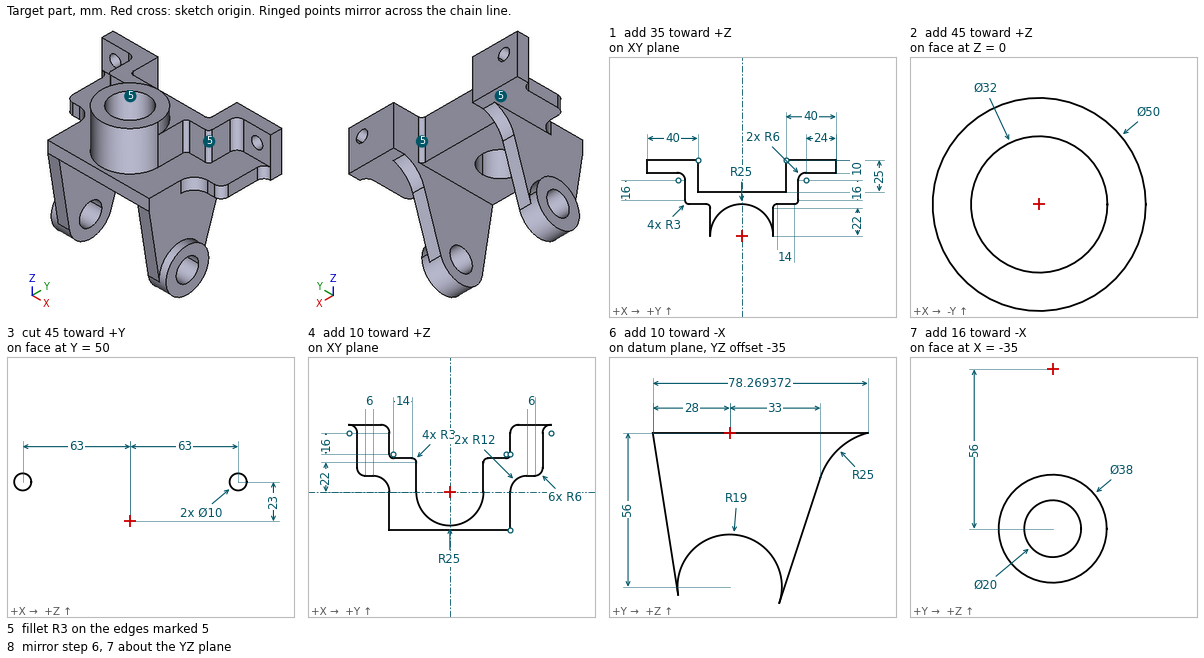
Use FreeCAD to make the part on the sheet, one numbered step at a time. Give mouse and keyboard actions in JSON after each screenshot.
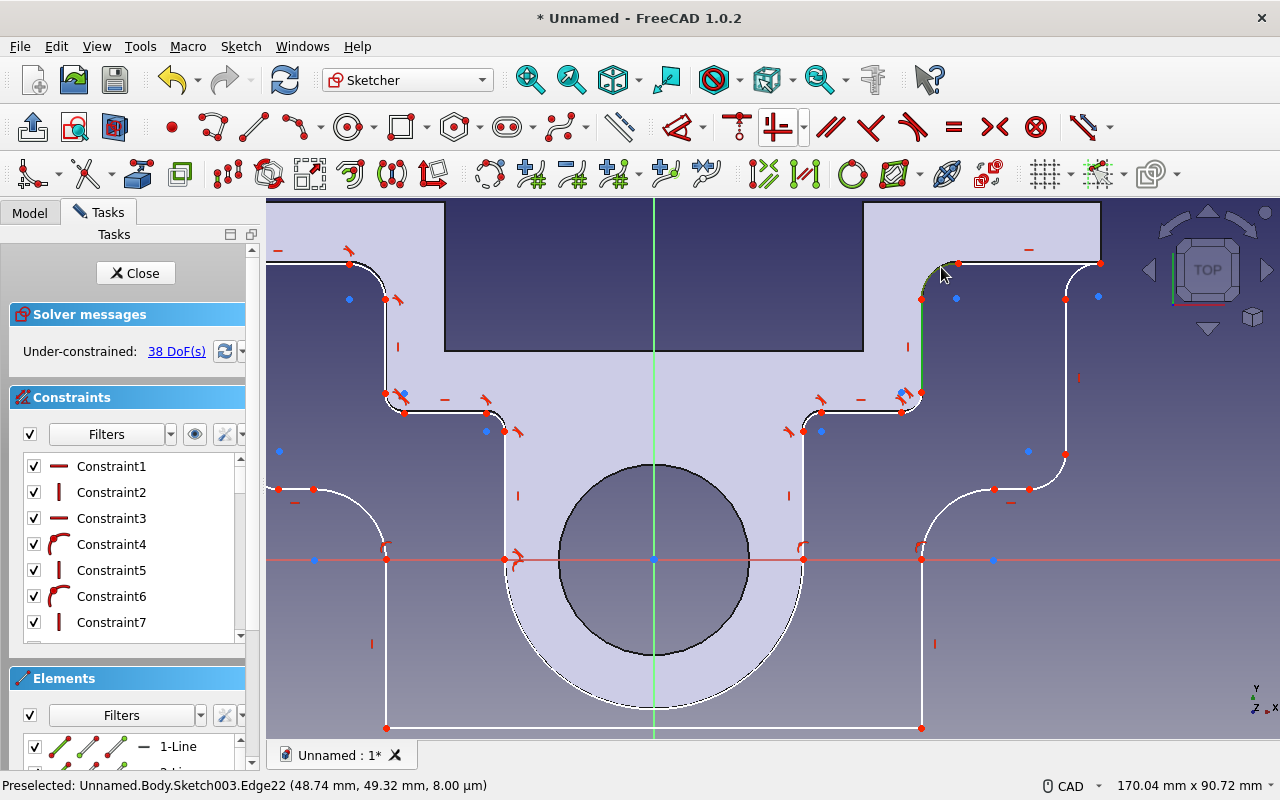
{"action": "left_click", "coordinate": [913, 128]}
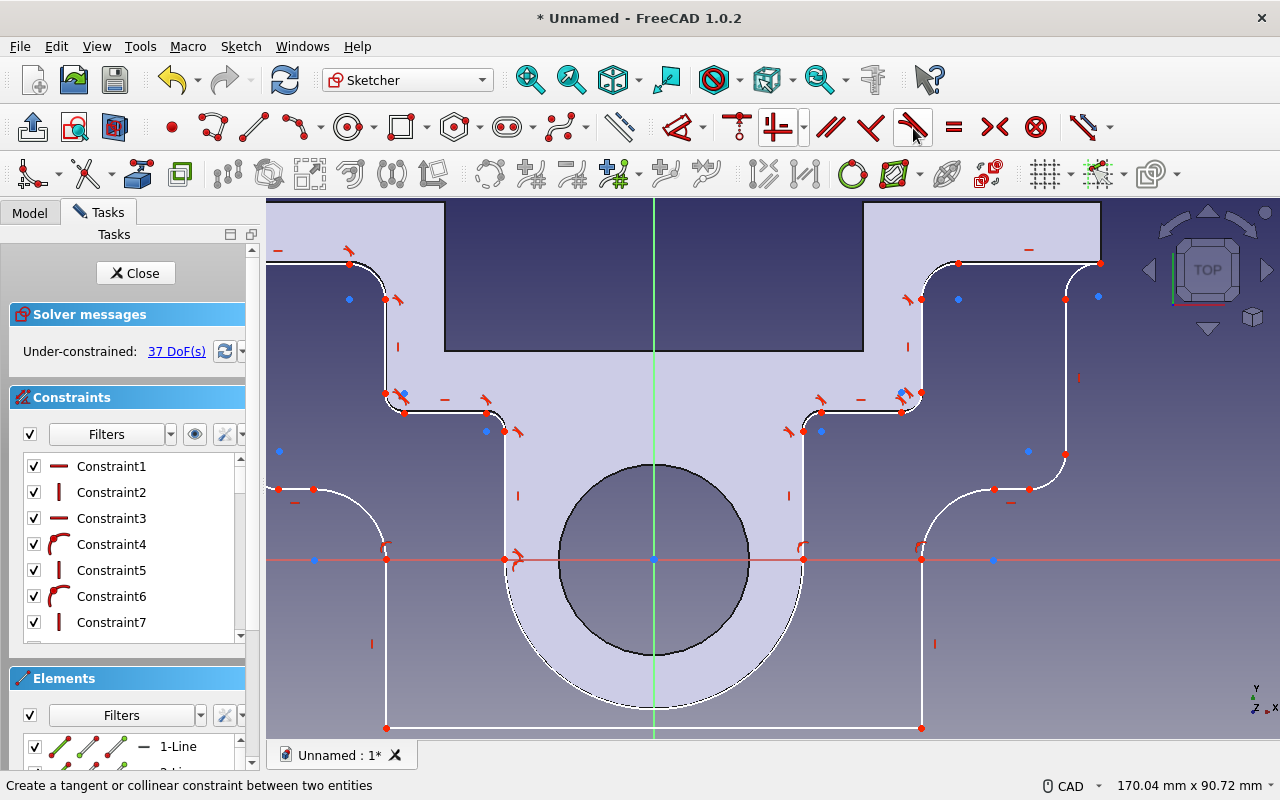
{"action": "left_click", "coordinate": [1001, 264]}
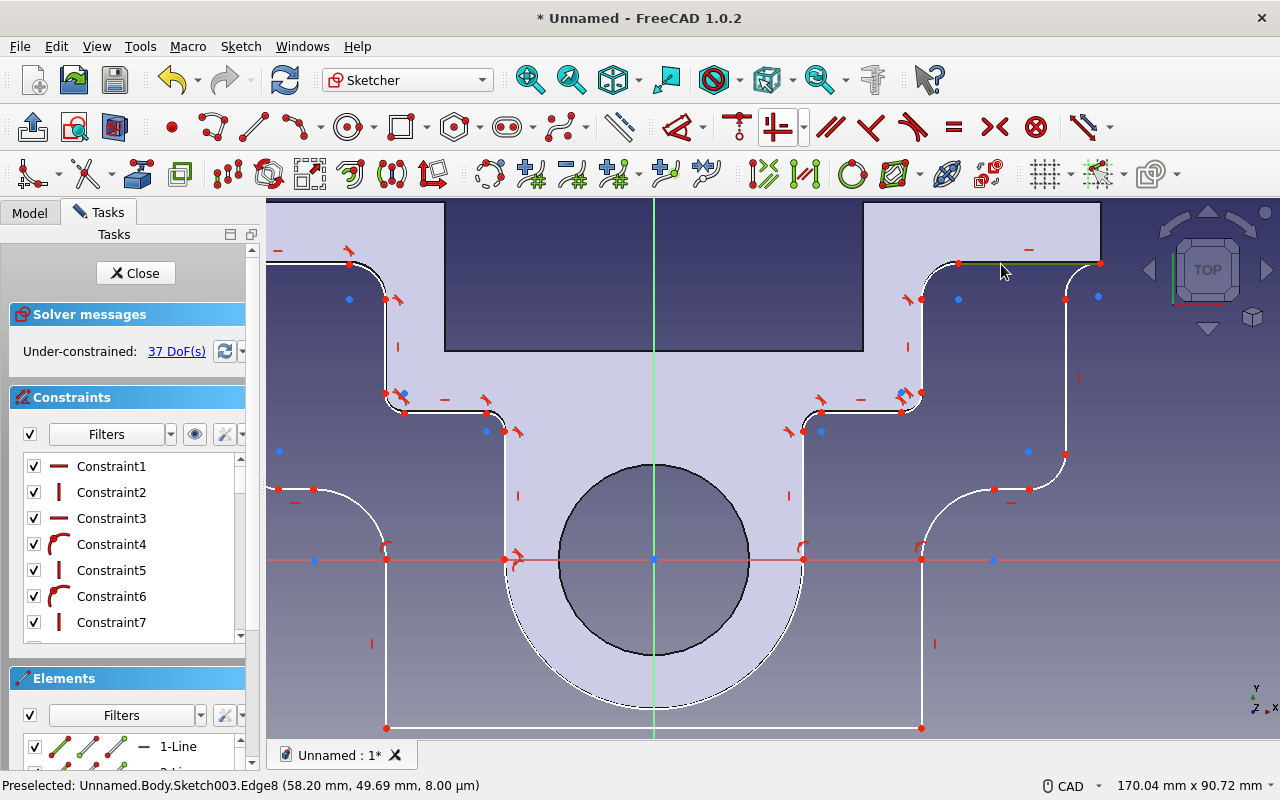
{"action": "left_click", "coordinate": [942, 267]}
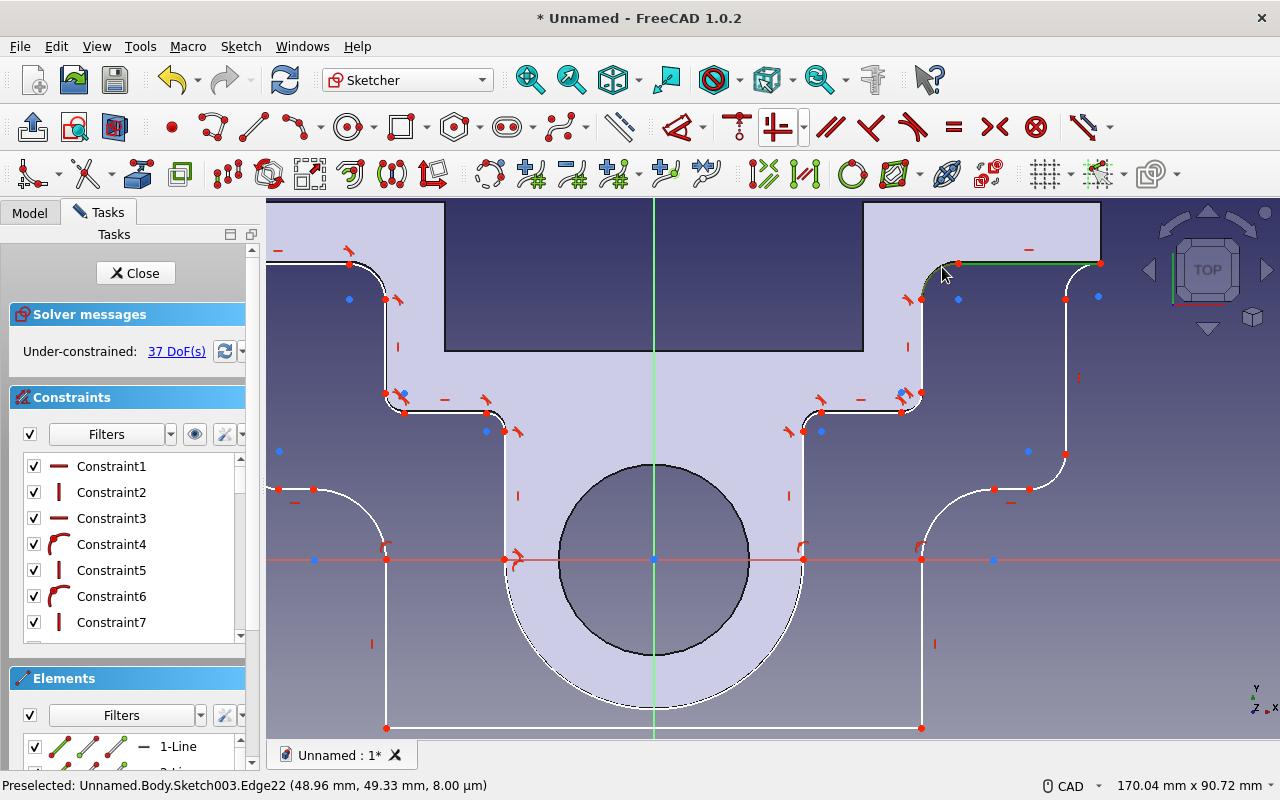
{"action": "left_click", "coordinate": [913, 128]}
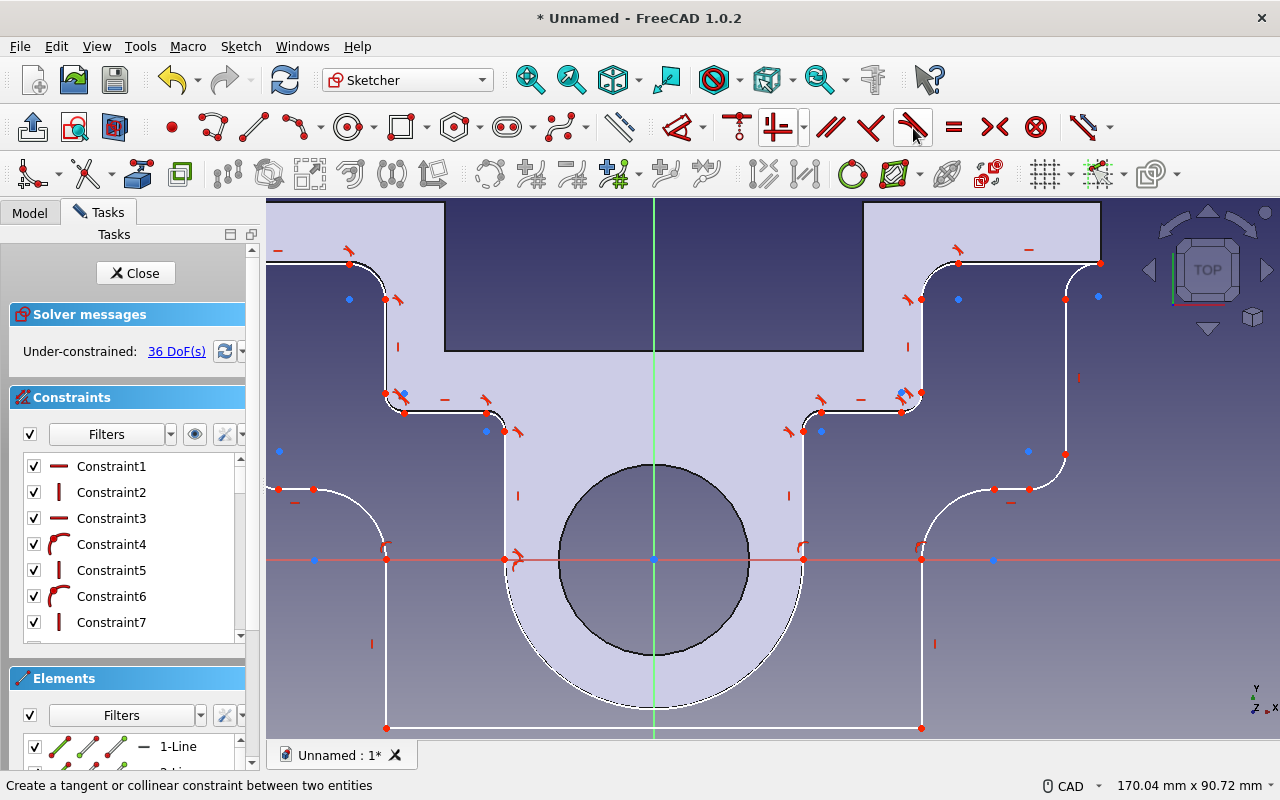
{"action": "left_click", "coordinate": [1001, 264]}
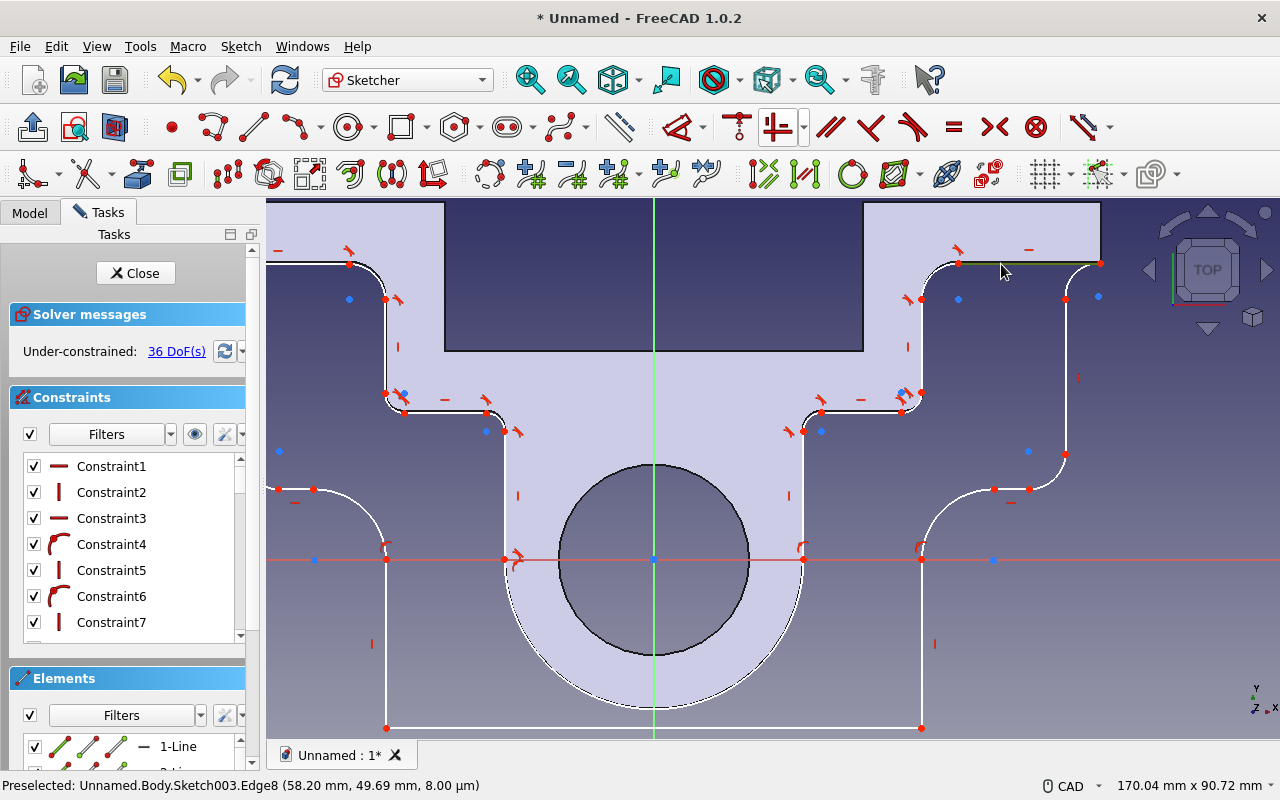
{"action": "left_click", "coordinate": [1068, 283]}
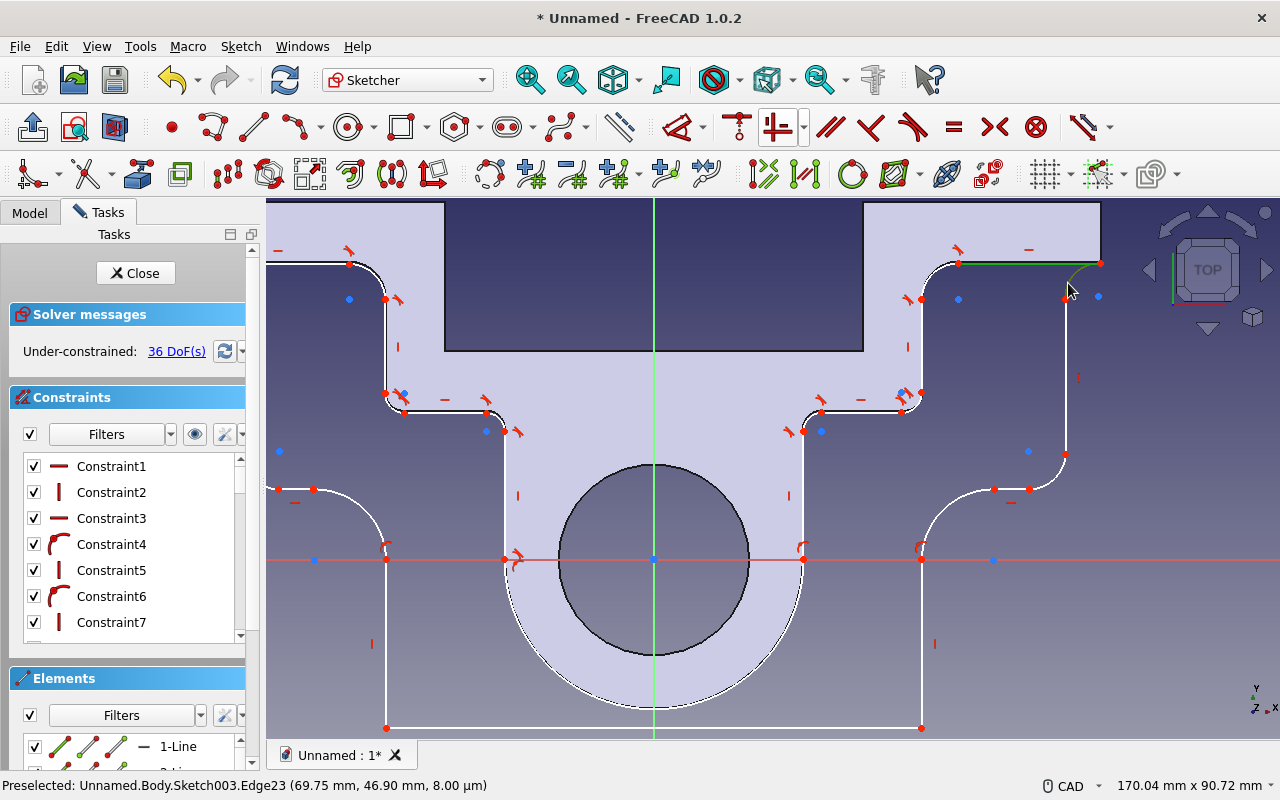
{"action": "left_click", "coordinate": [913, 128]}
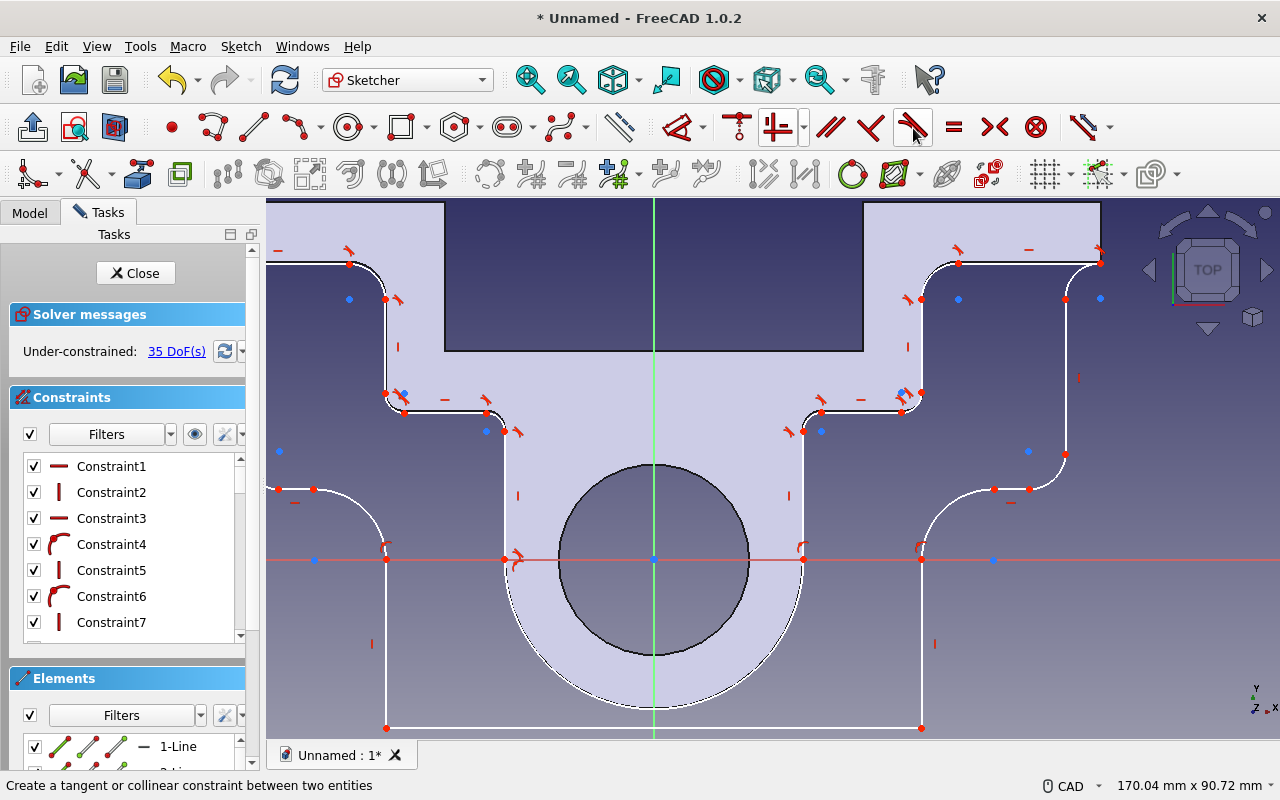
{"action": "left_click", "coordinate": [1066, 346]}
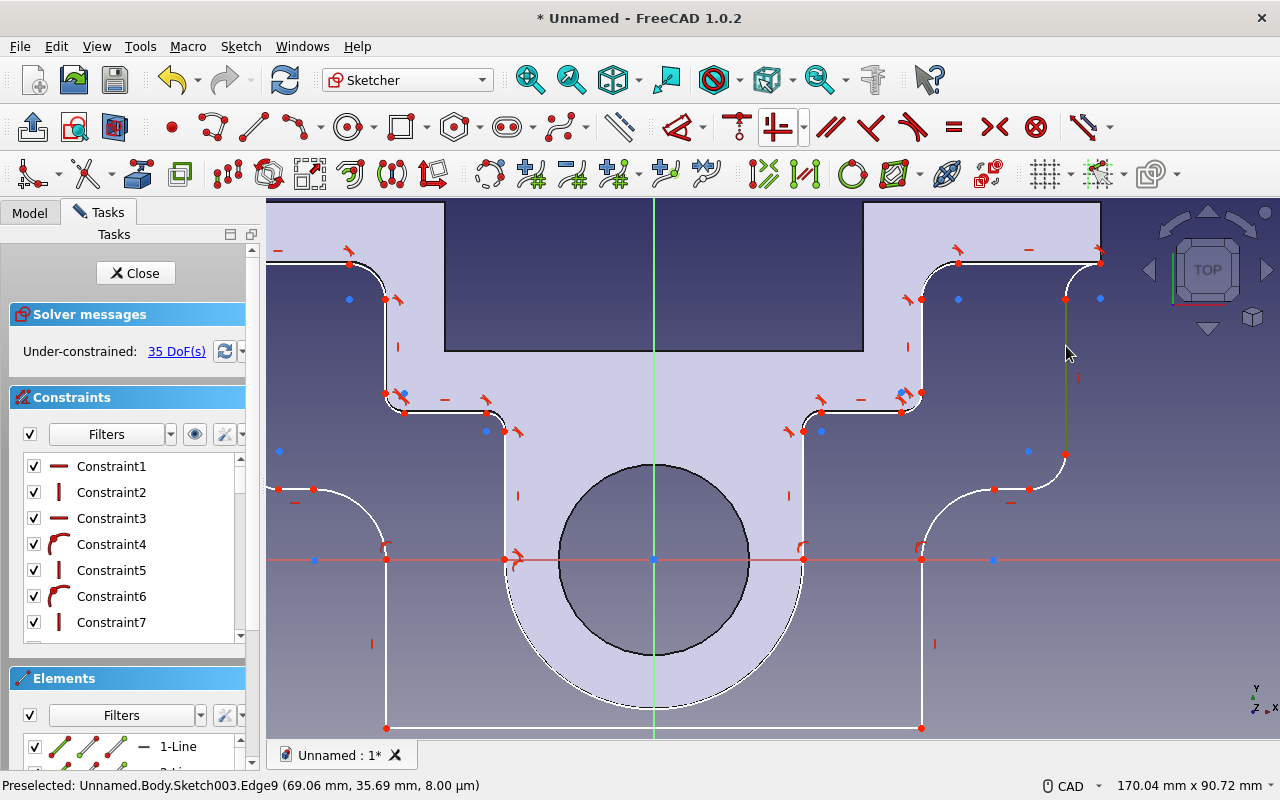
{"action": "left_click", "coordinate": [1069, 284]}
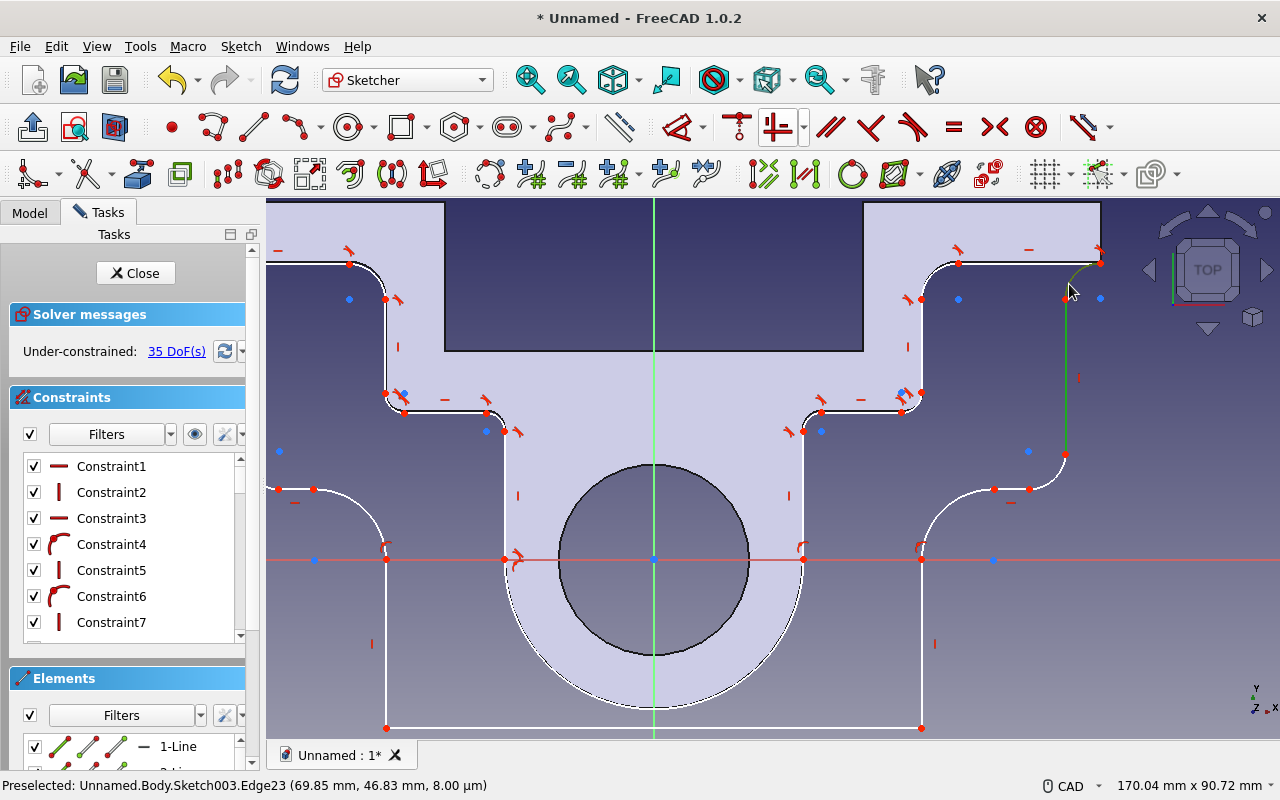
{"action": "left_click", "coordinate": [913, 128]}